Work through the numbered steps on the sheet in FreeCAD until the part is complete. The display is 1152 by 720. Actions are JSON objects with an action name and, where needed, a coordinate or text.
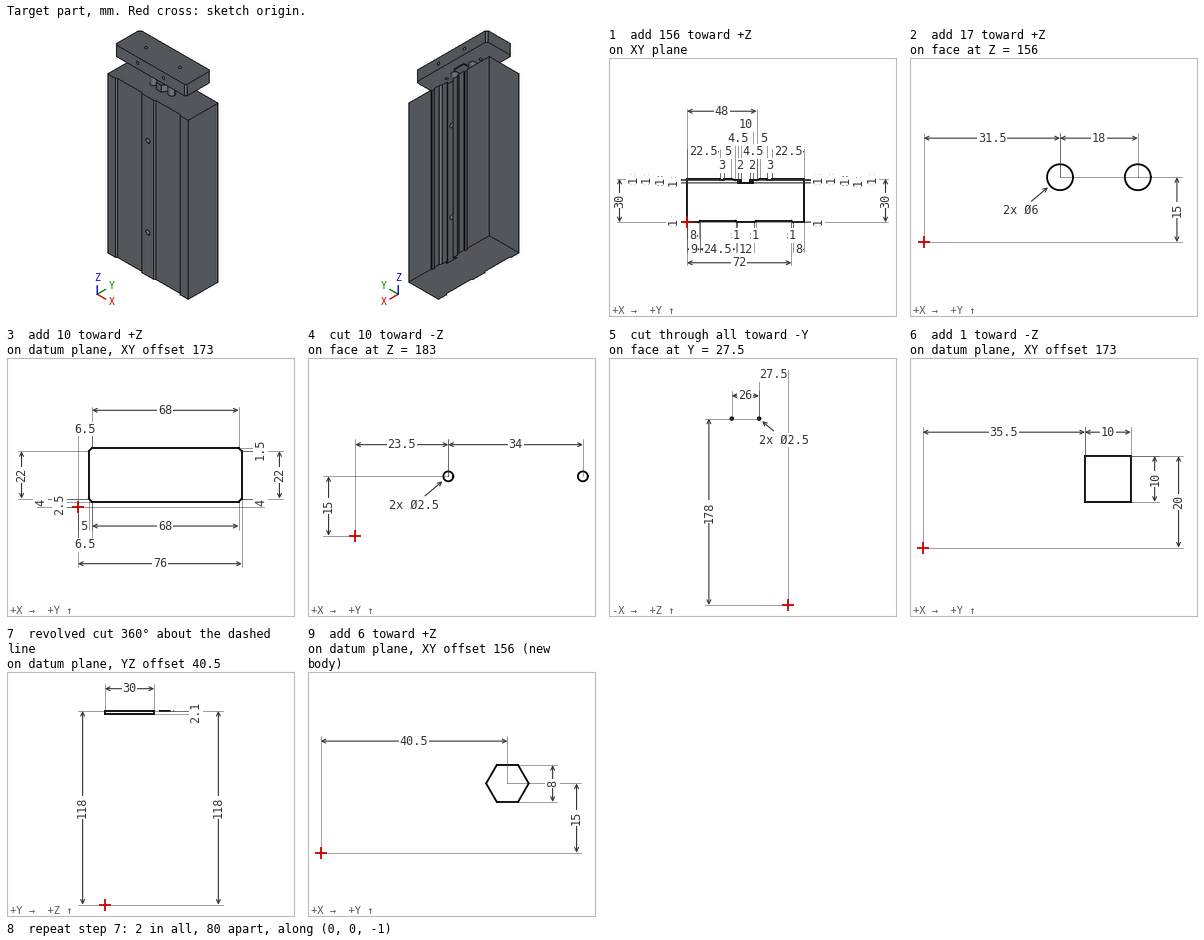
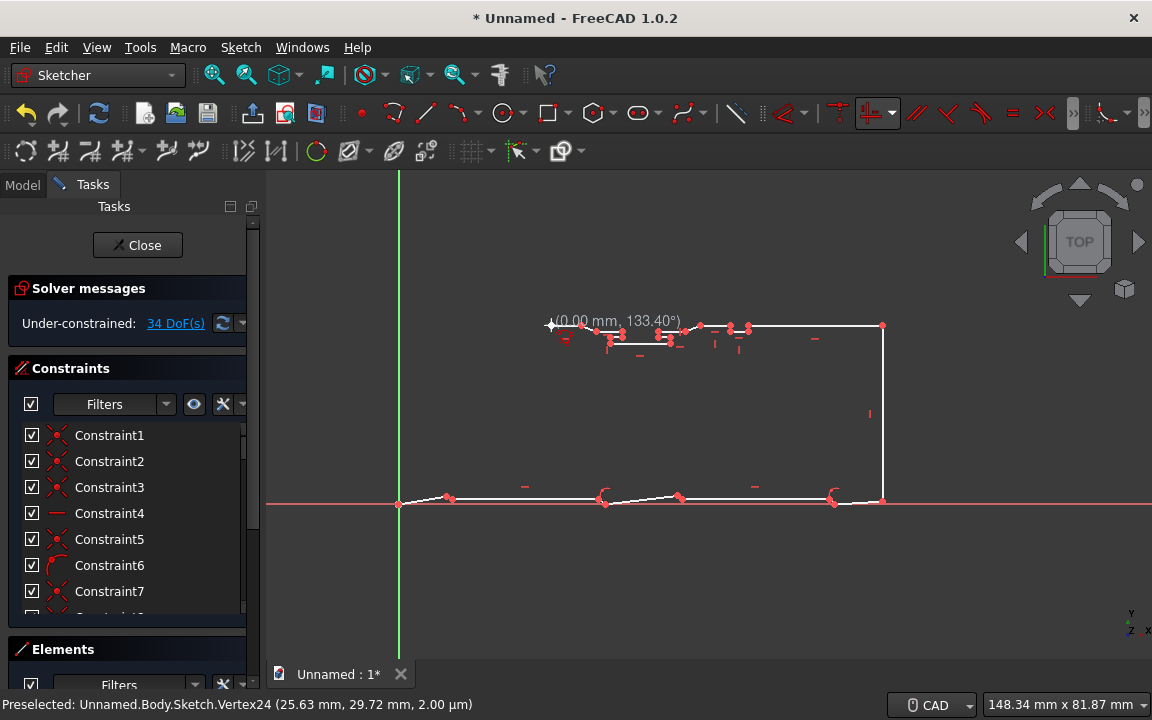
{"action": "scroll", "coordinate": [551, 331], "scroll_direction": "up", "scroll_amount": 5}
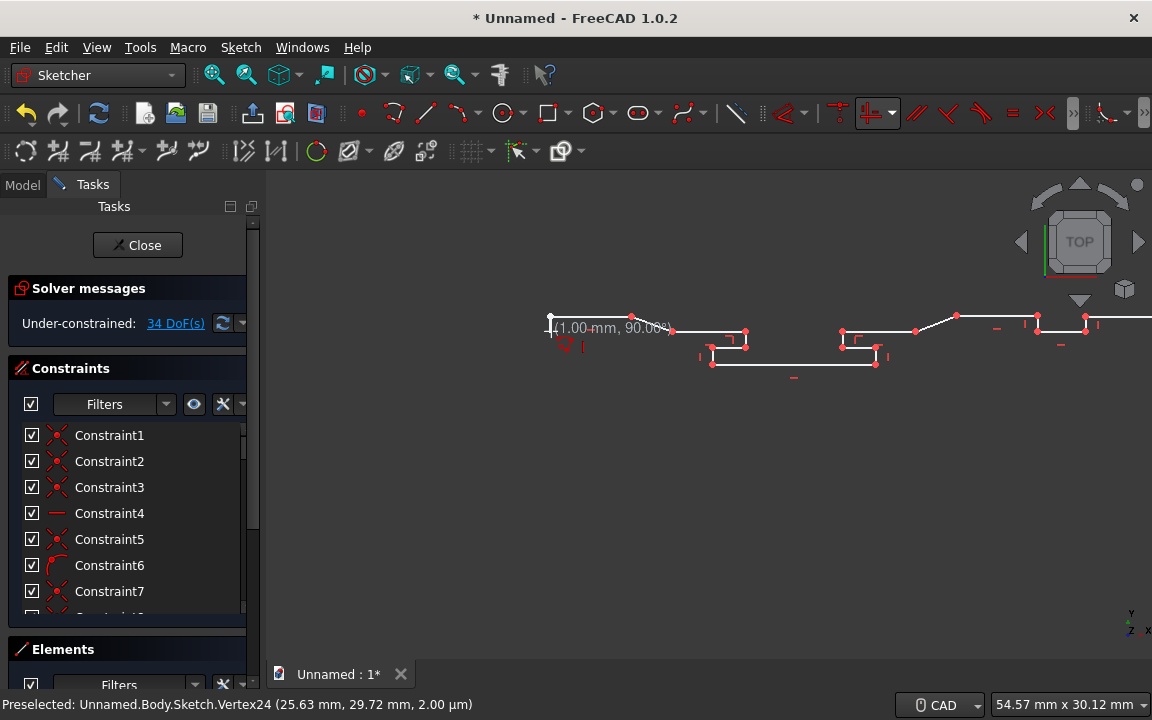
{"action": "left_click", "coordinate": [550, 331]}
{"action": "left_click", "coordinate": [502, 331]}
{"action": "left_click", "coordinate": [502, 315]}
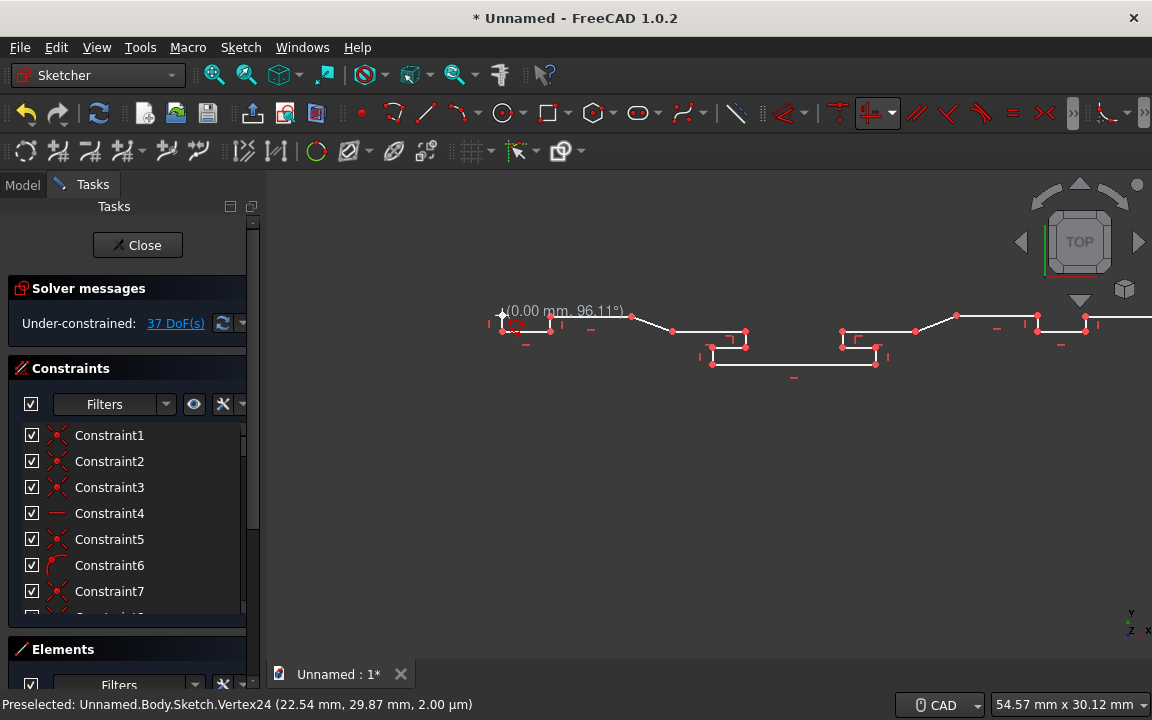
{"action": "scroll", "coordinate": [551, 331], "scroll_direction": "down", "scroll_amount": 5}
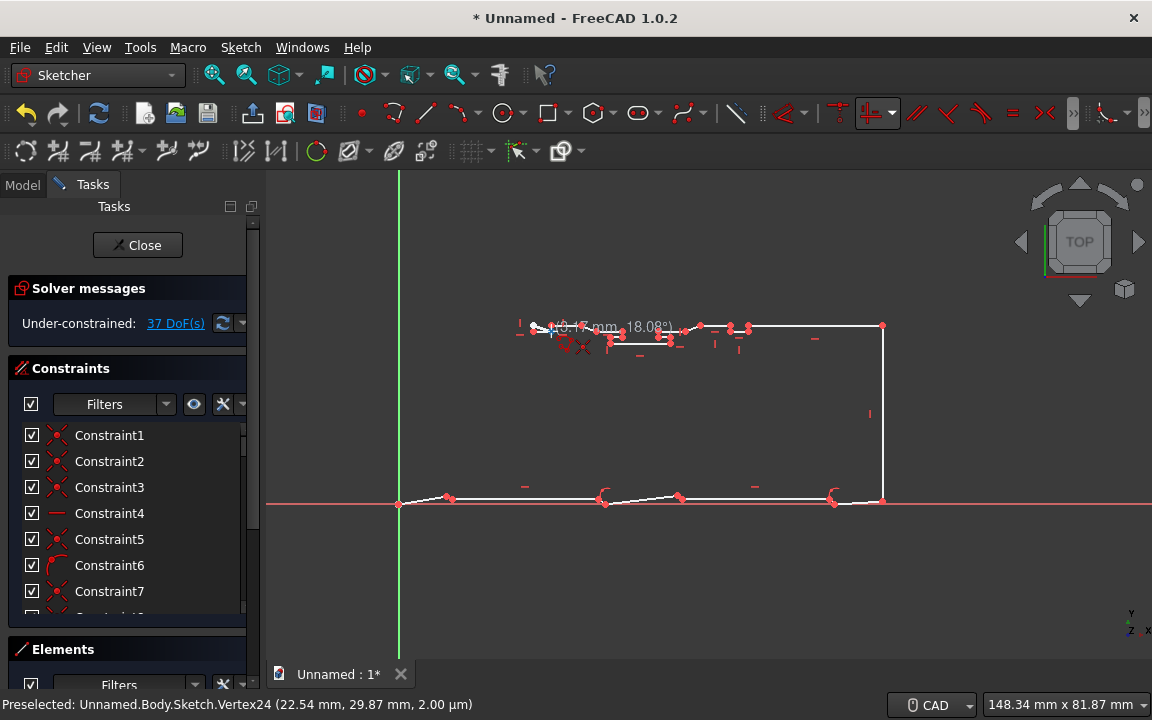
{"action": "left_click", "coordinate": [408, 325]}
{"action": "left_click", "coordinate": [399, 504]}
{"action": "key", "text": "Escape"}
{"action": "key", "text": "Escape"}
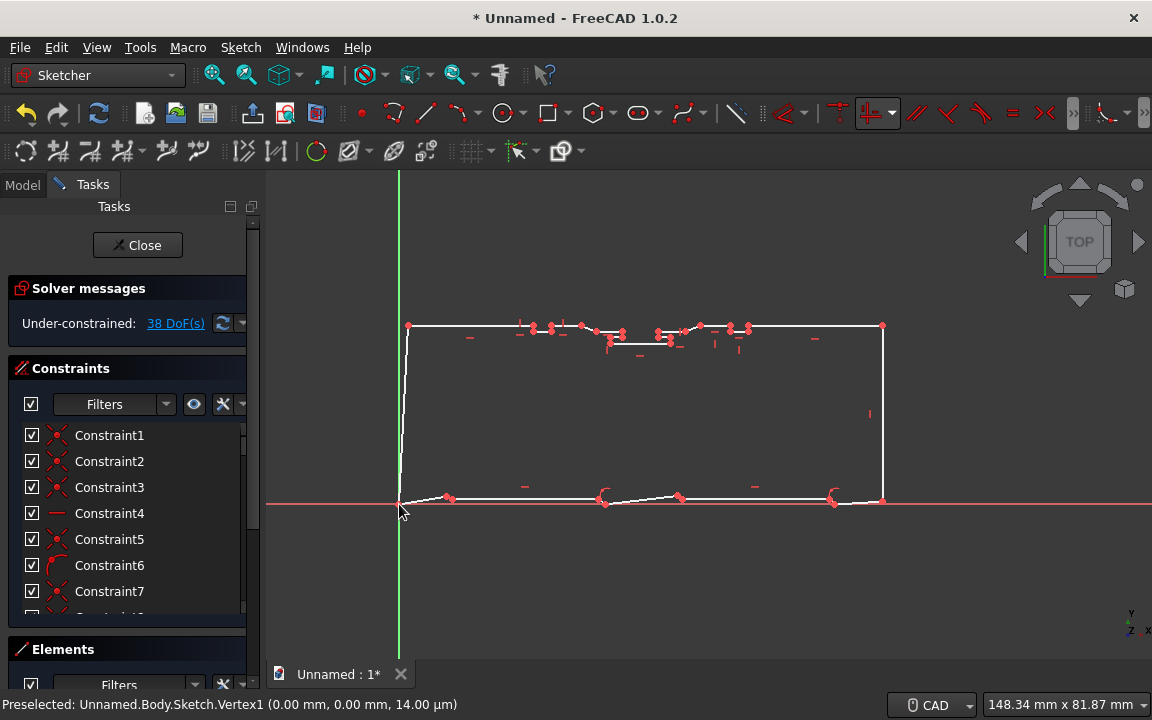
{"action": "left_click", "coordinate": [413, 502]}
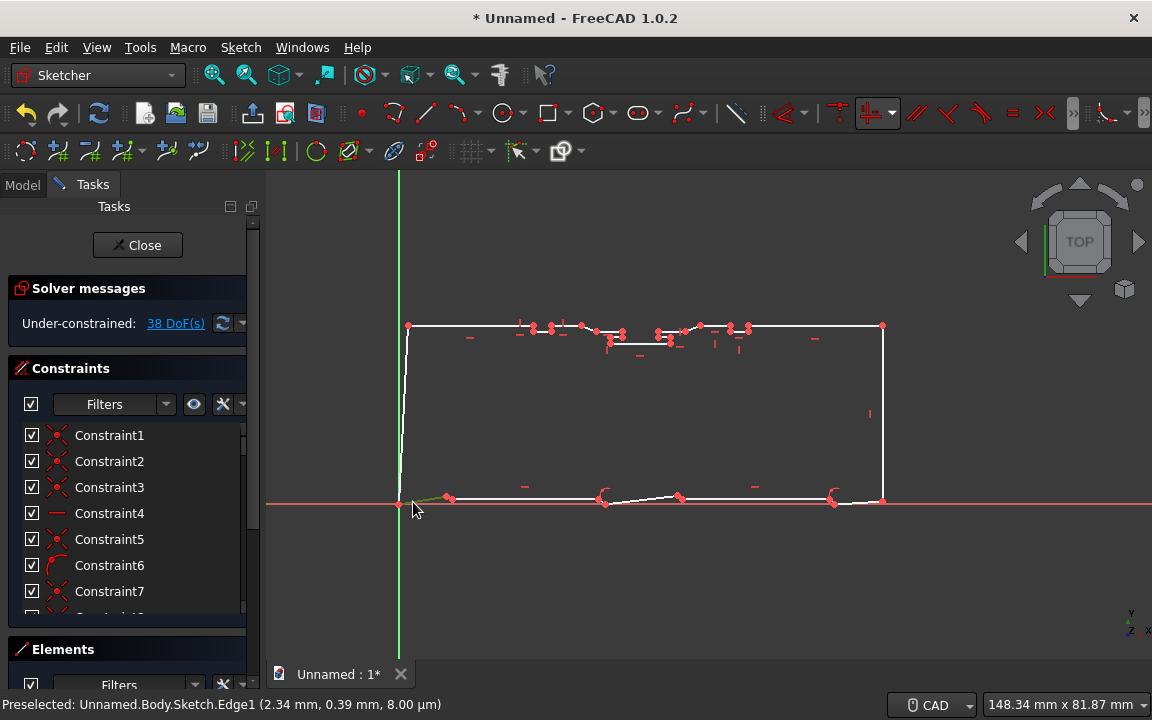
{"action": "key", "text": "h"}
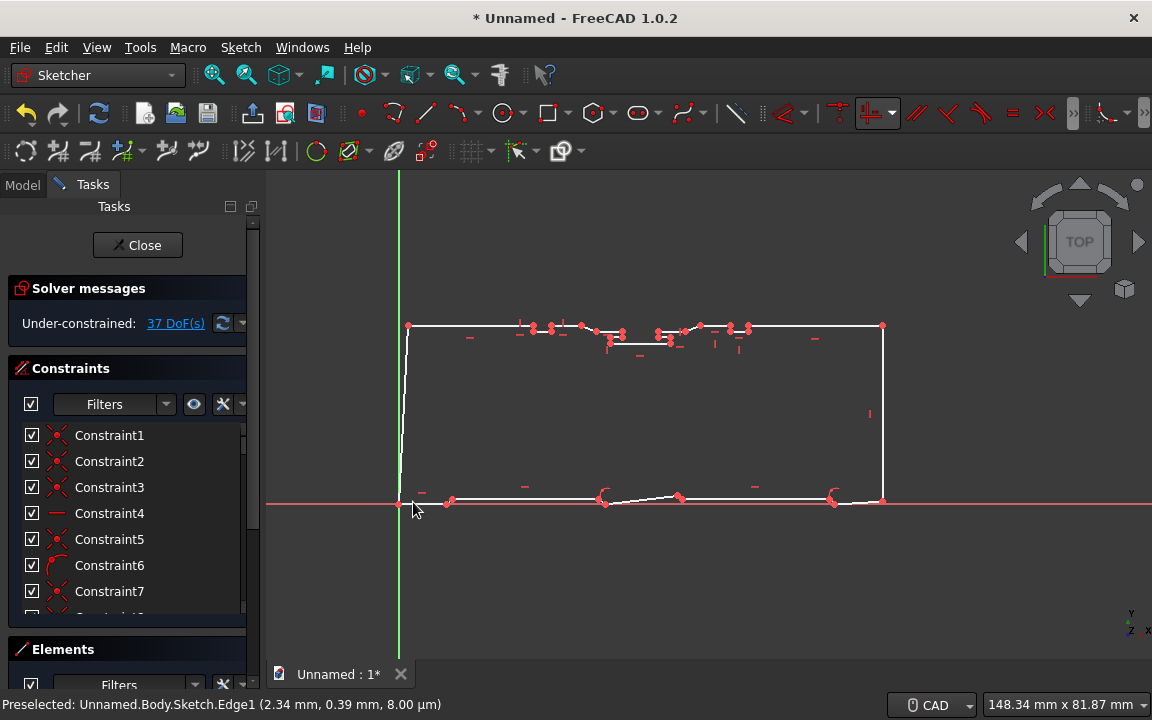
{"action": "left_click", "coordinate": [627, 502]}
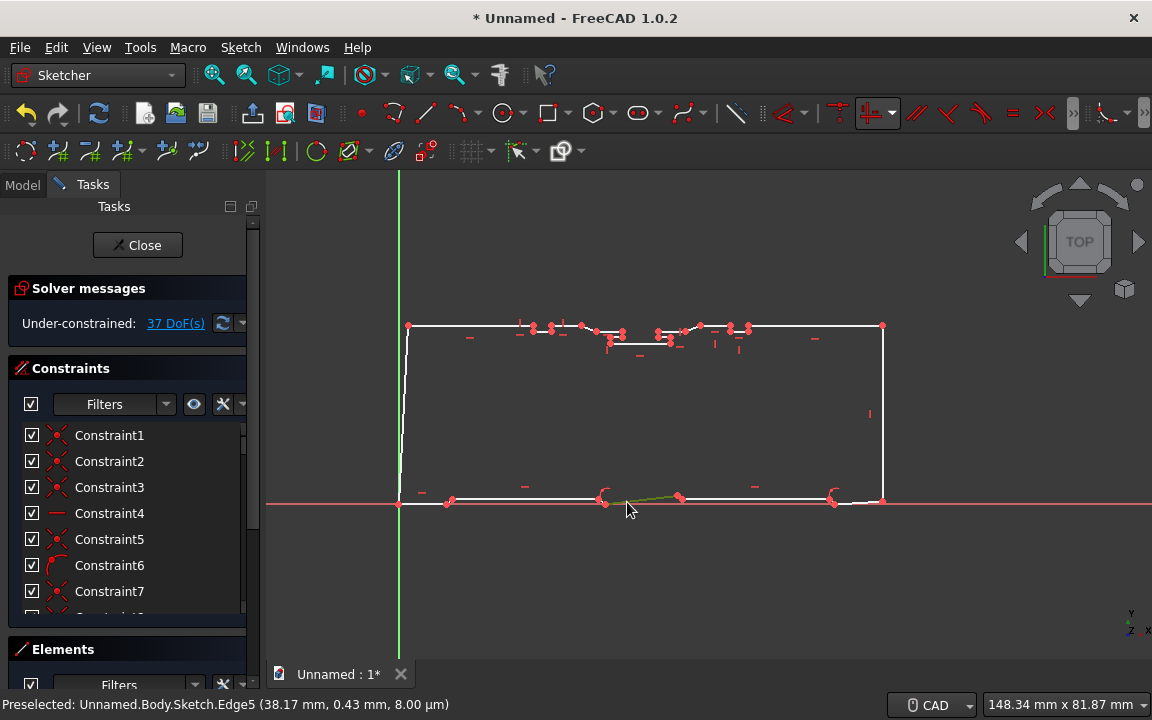
{"action": "left_click", "coordinate": [894, 114]}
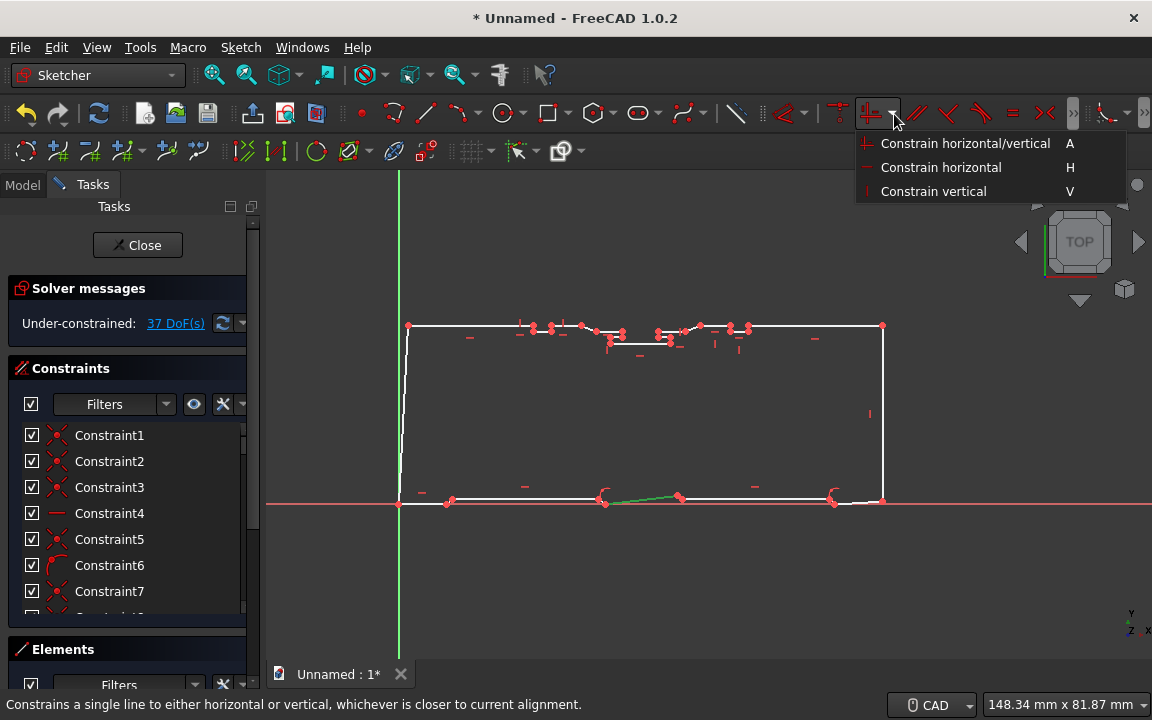
{"action": "left_click", "coordinate": [991, 167]}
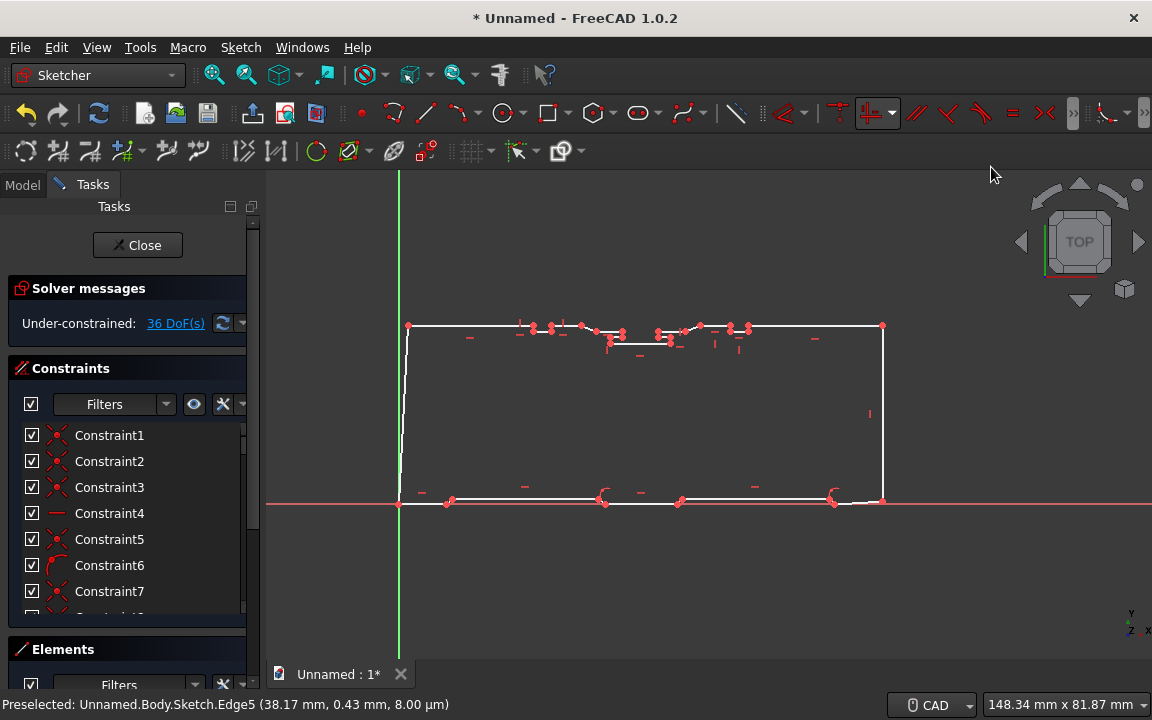
{"action": "left_click", "coordinate": [849, 504]}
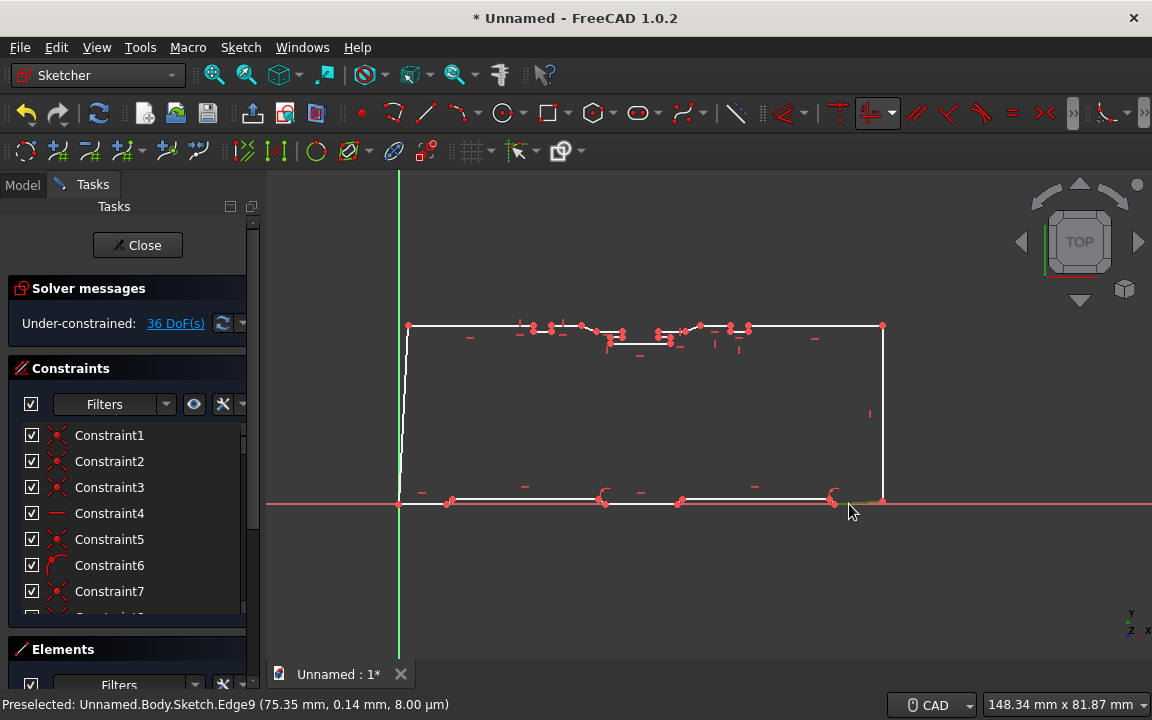
{"action": "key", "text": "h"}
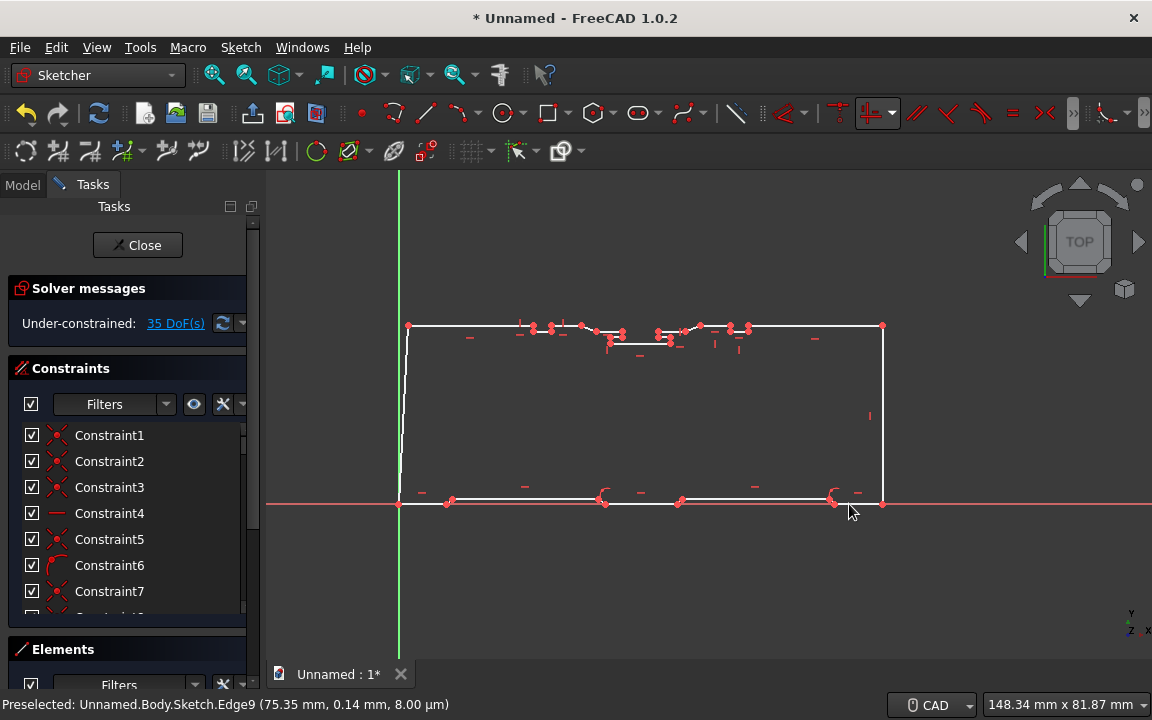
{"action": "left_click", "coordinate": [402, 451]}